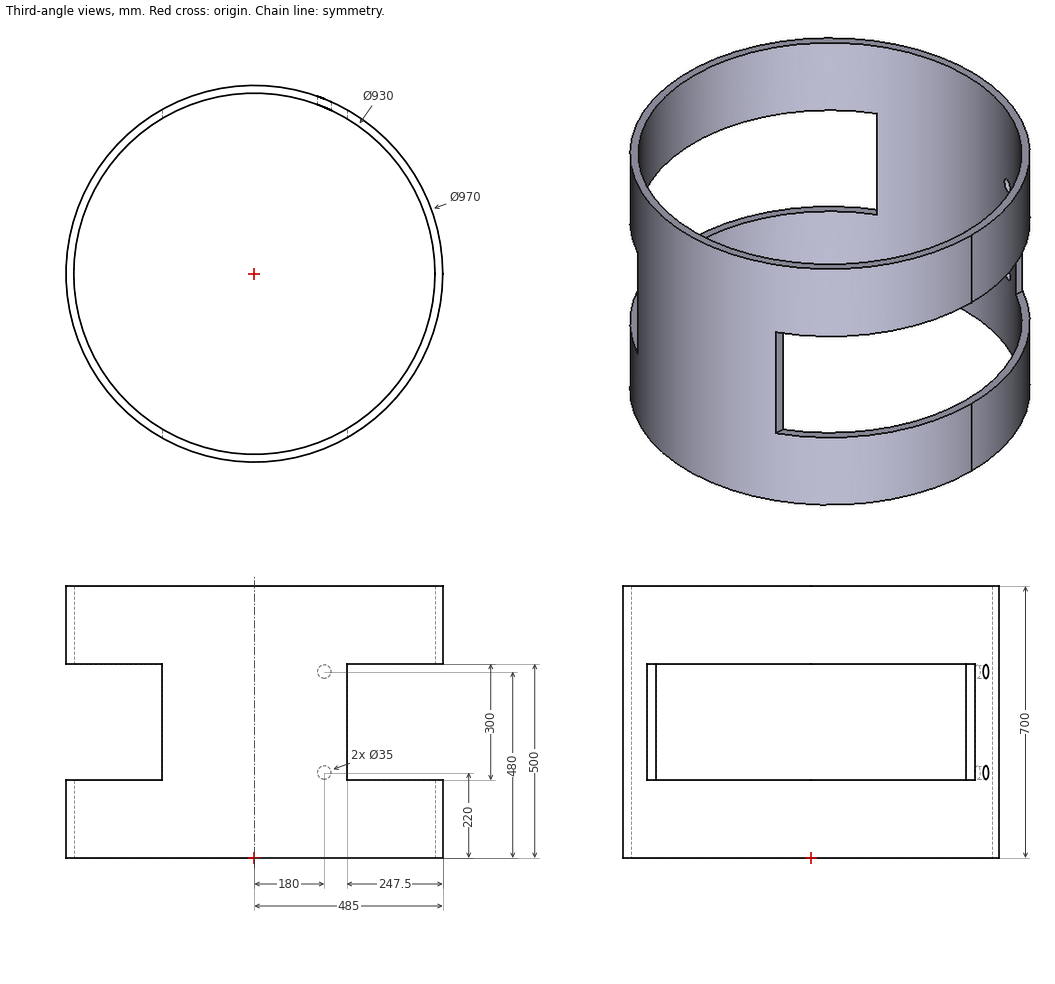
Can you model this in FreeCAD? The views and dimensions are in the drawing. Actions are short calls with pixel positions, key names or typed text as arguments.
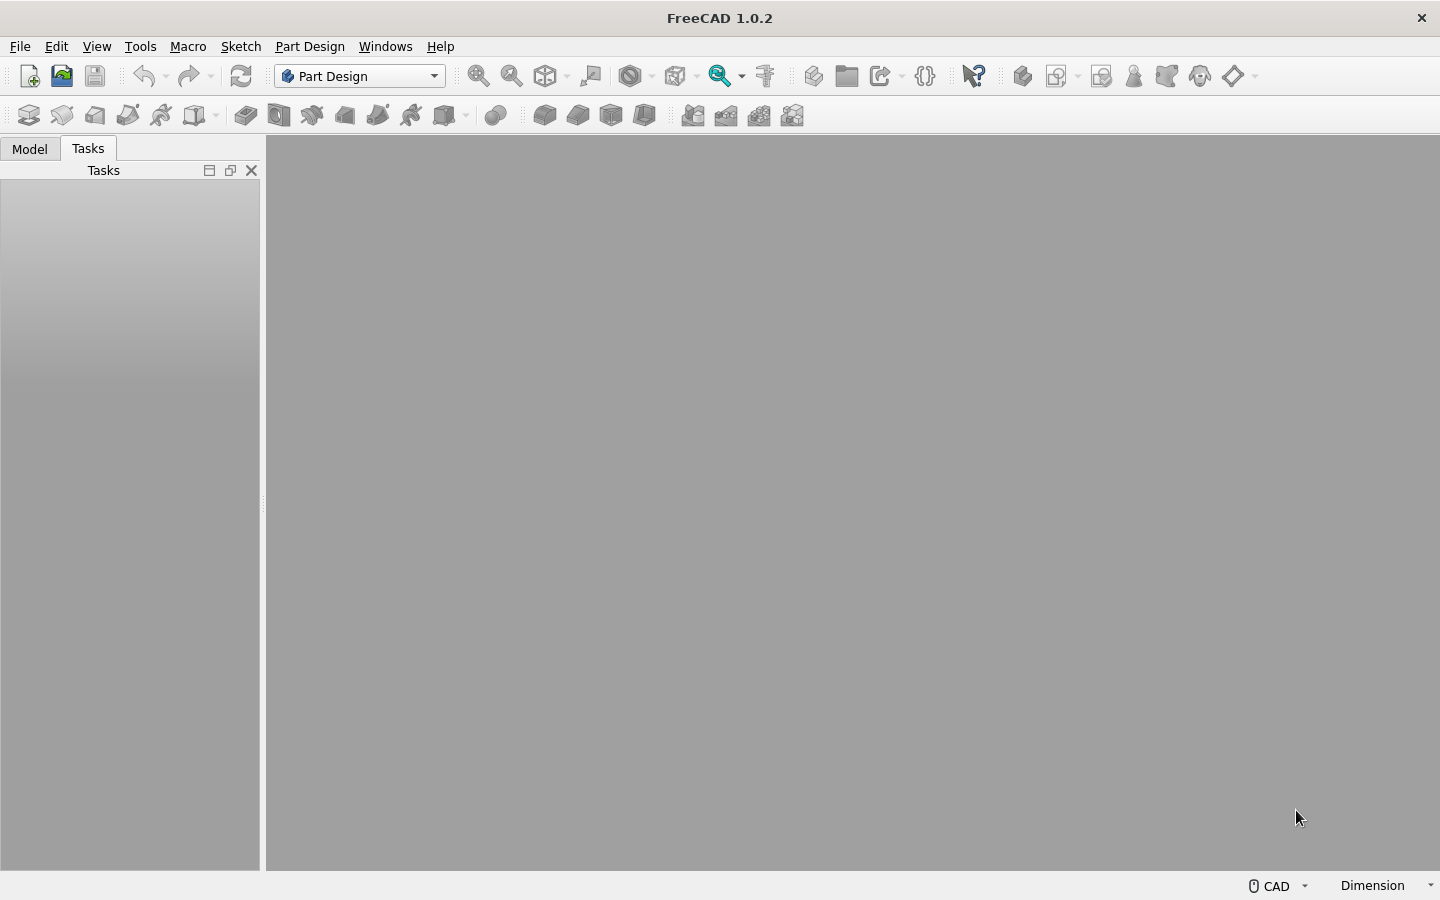
key(ctrl+n)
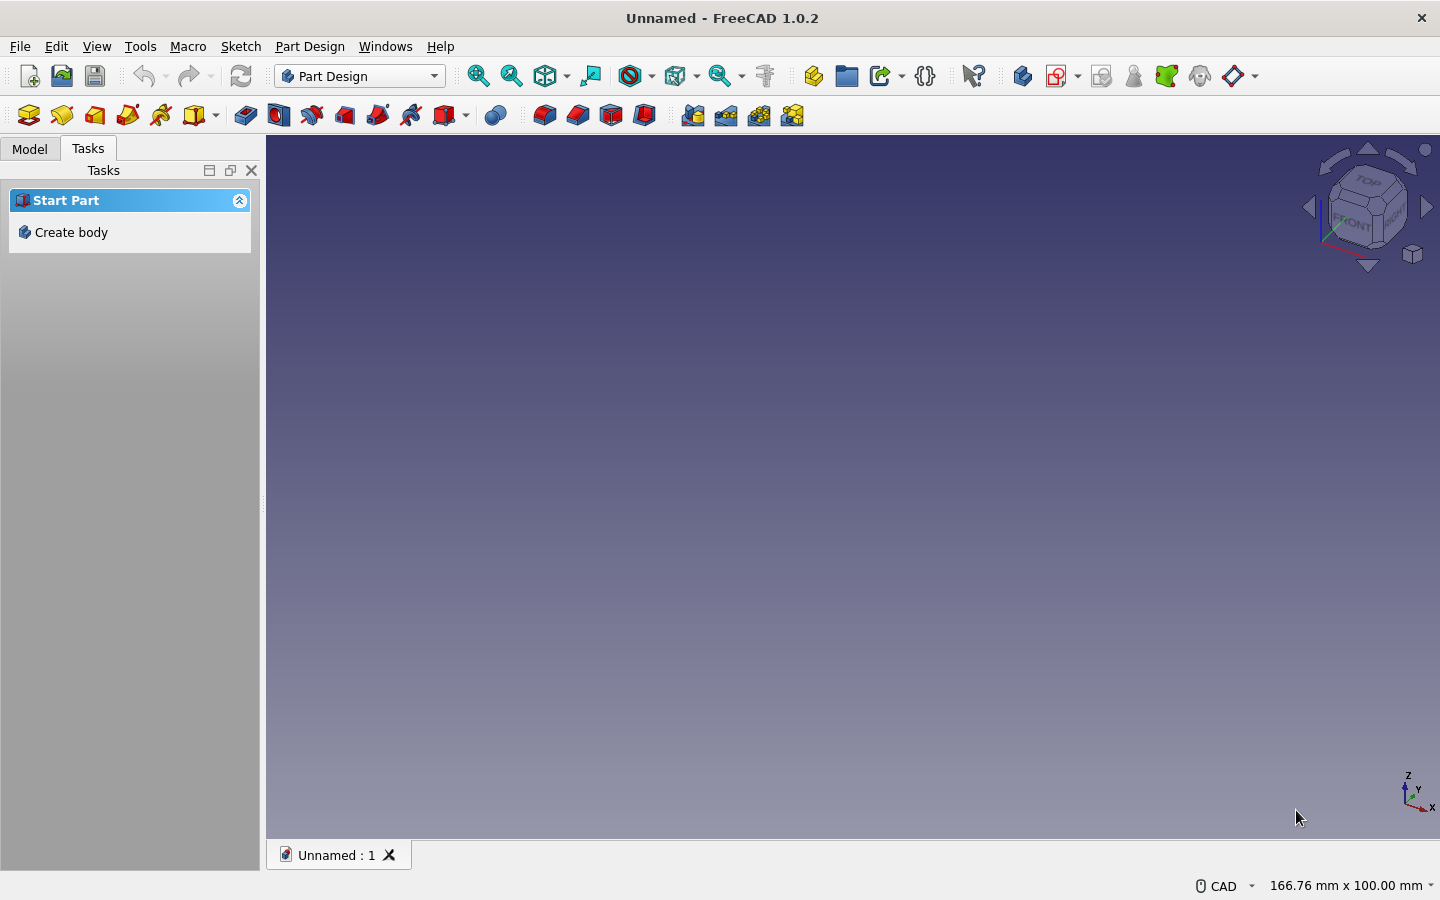
click(1056, 76)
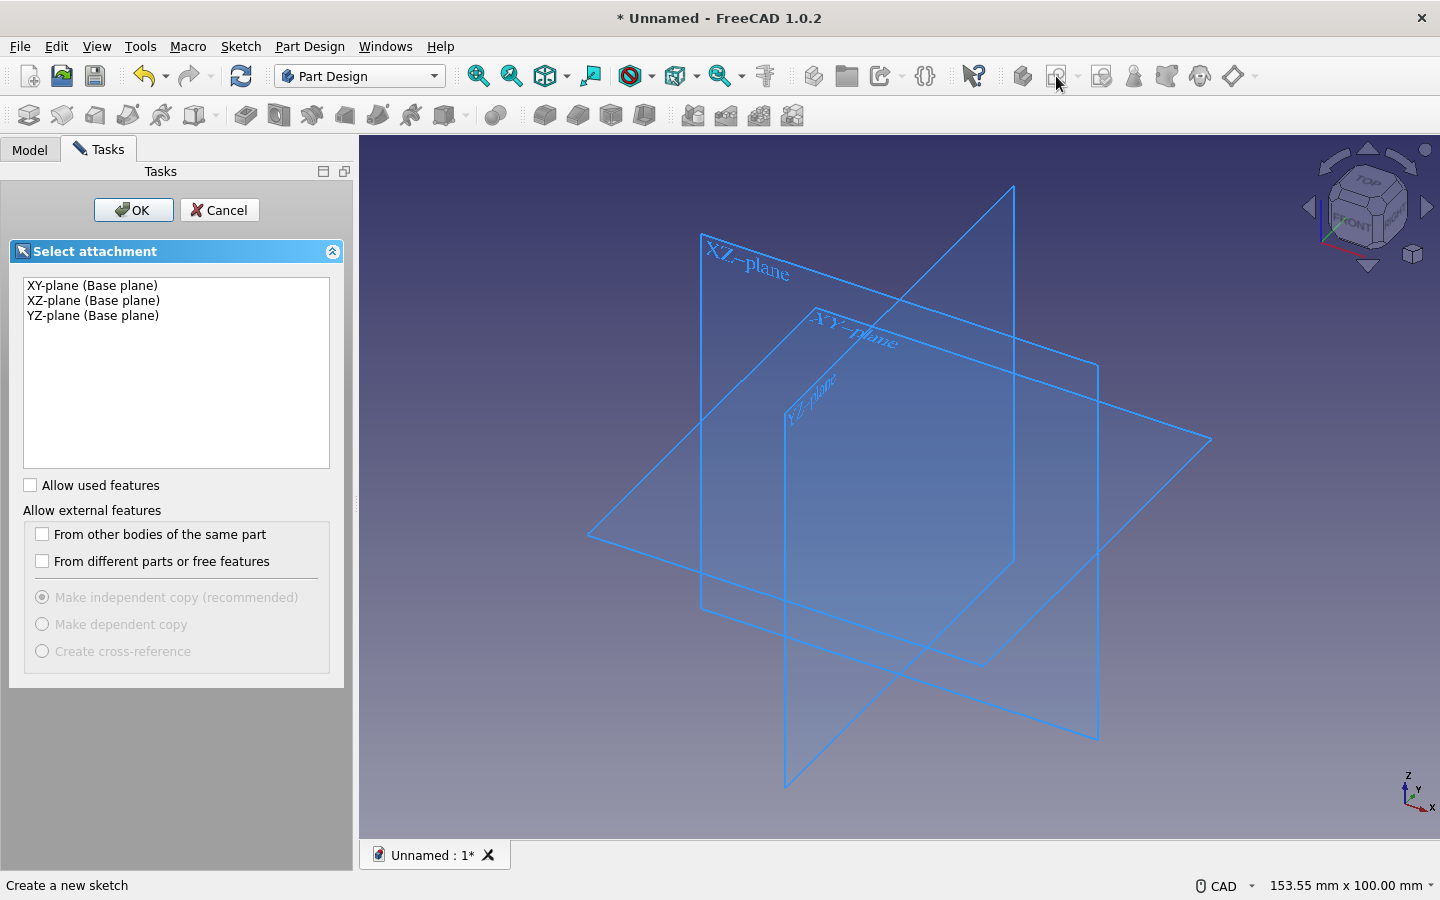
click(84, 286)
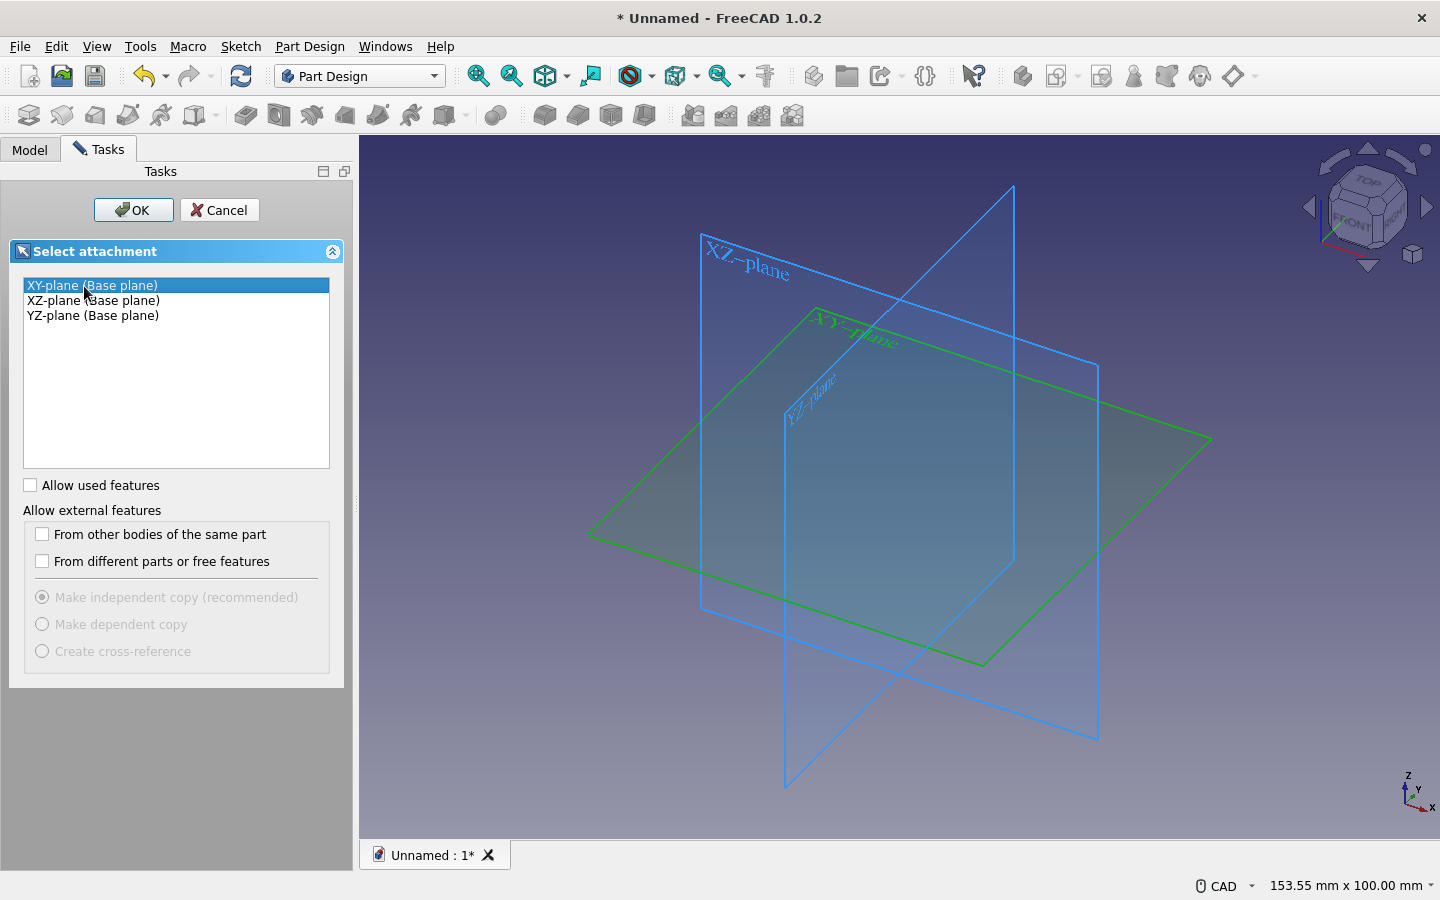
click(134, 210)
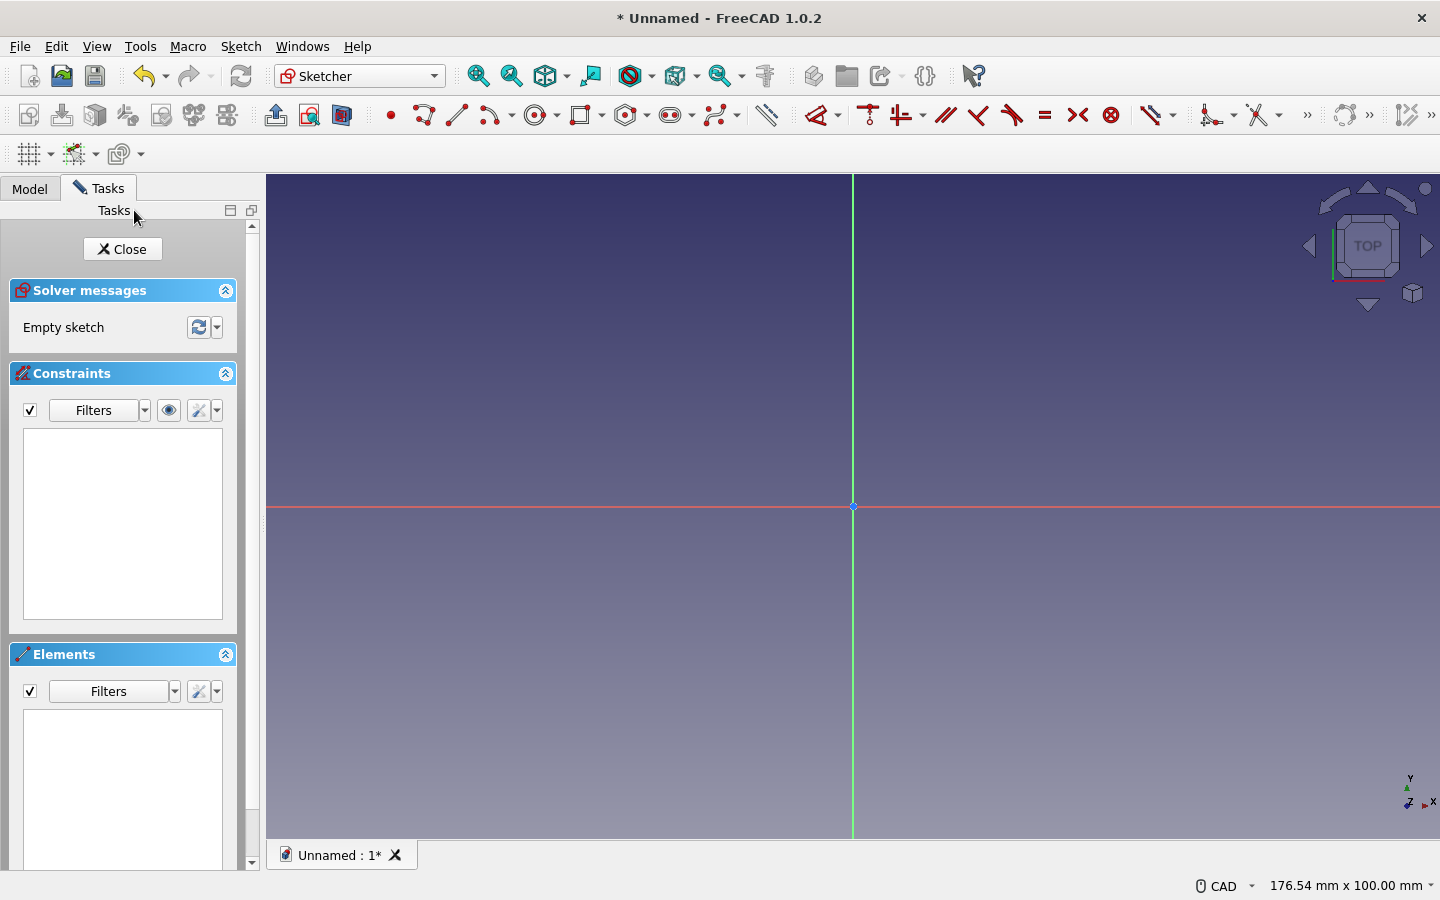
scroll(780, 506, down, 14)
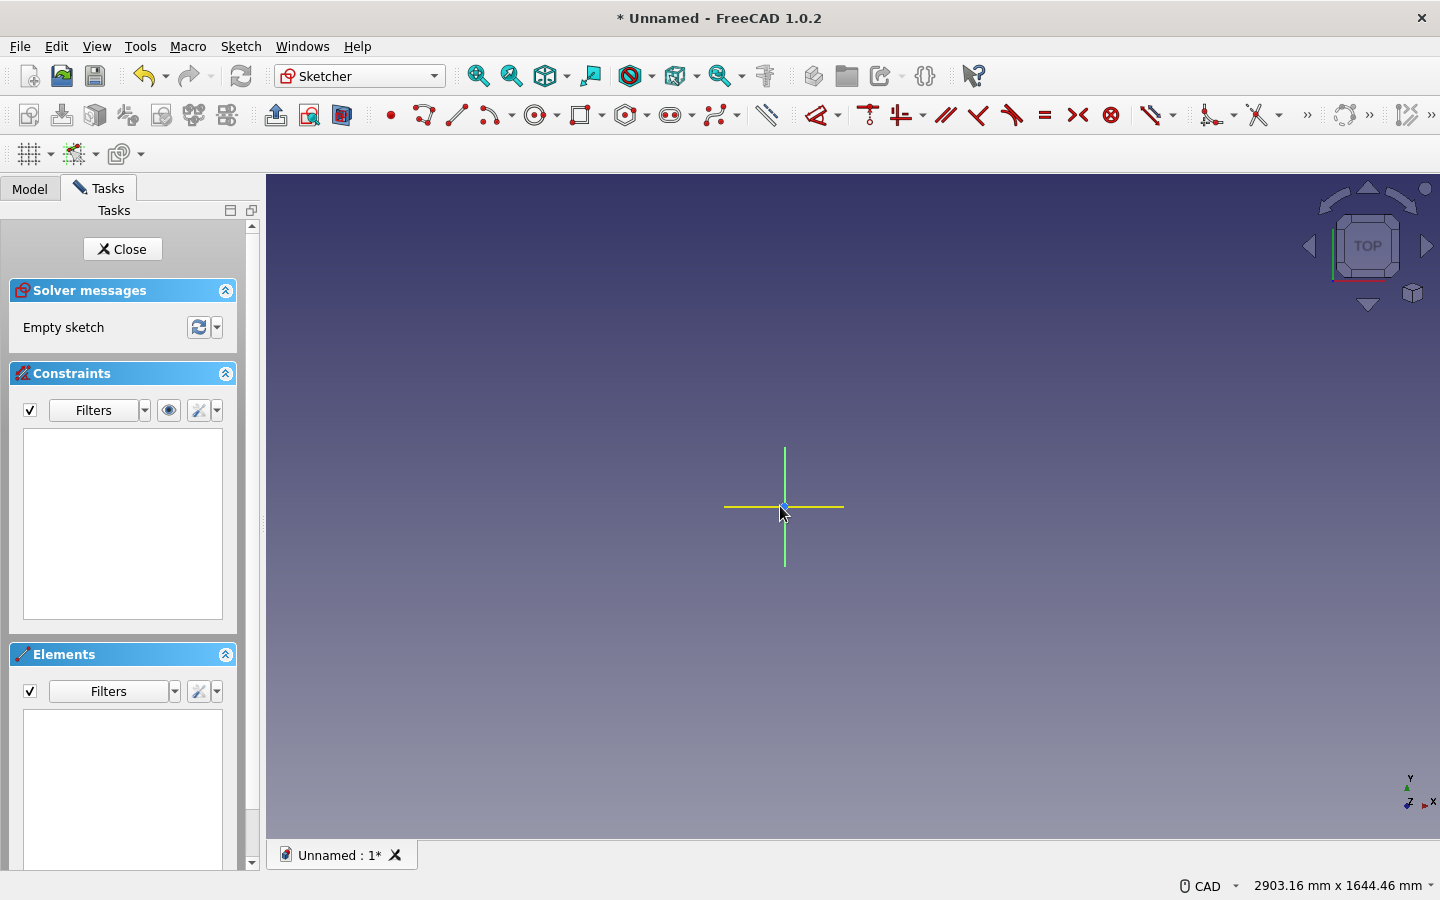
click(534, 116)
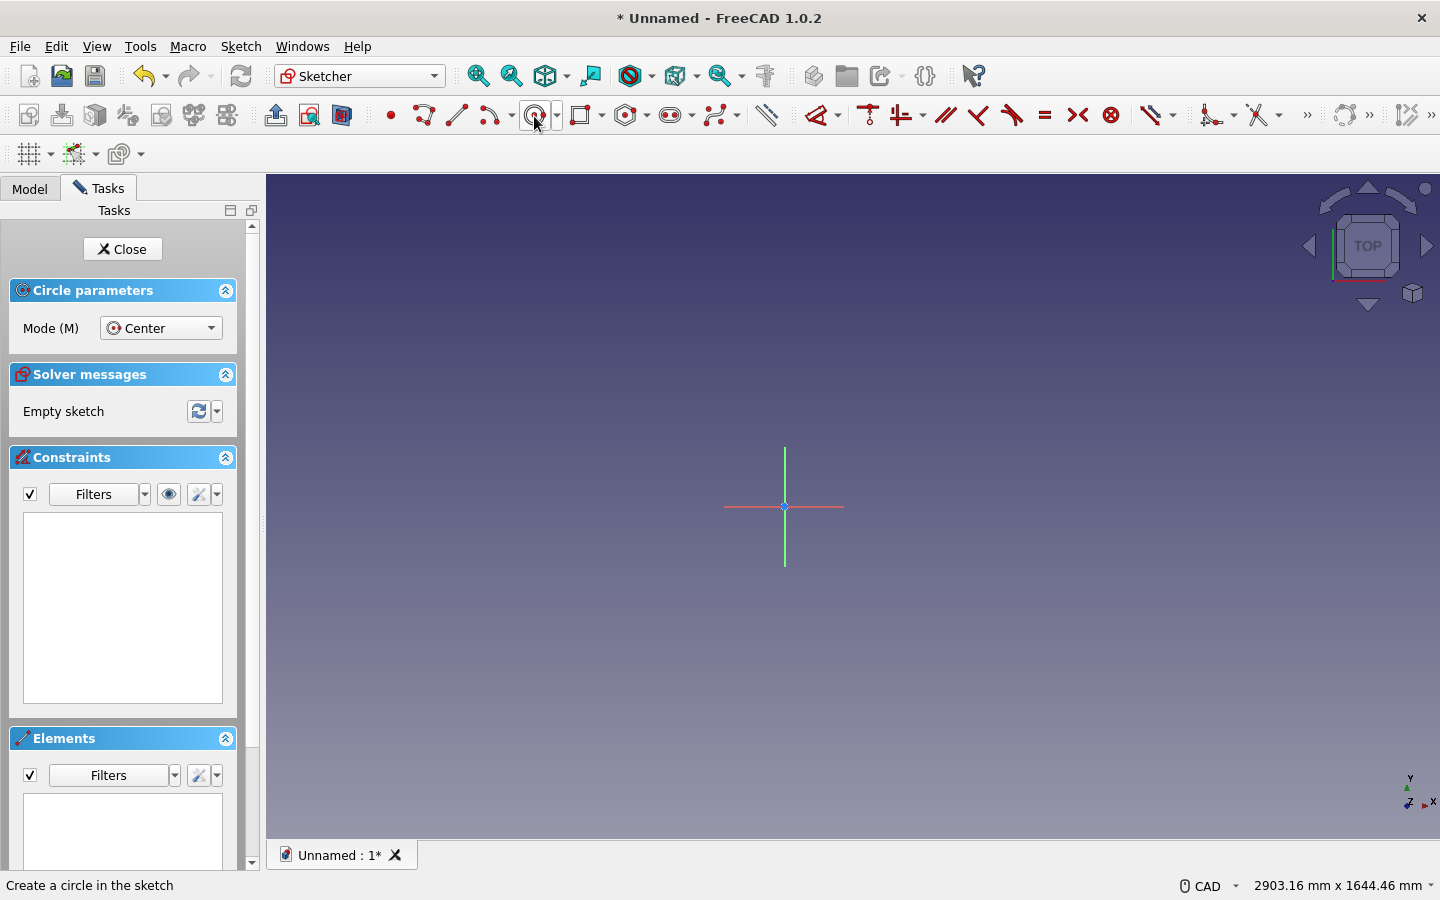
click(785, 506)
click(924, 368)